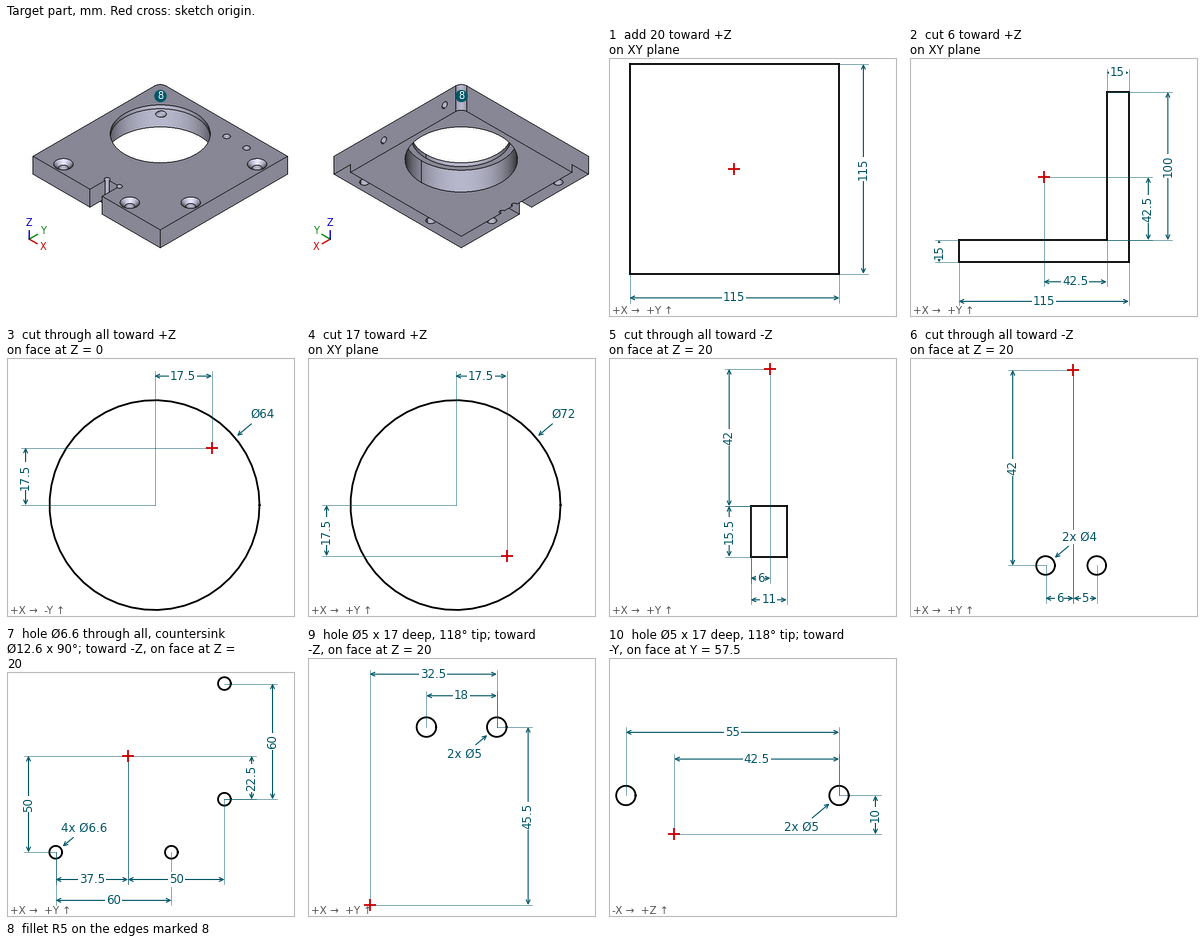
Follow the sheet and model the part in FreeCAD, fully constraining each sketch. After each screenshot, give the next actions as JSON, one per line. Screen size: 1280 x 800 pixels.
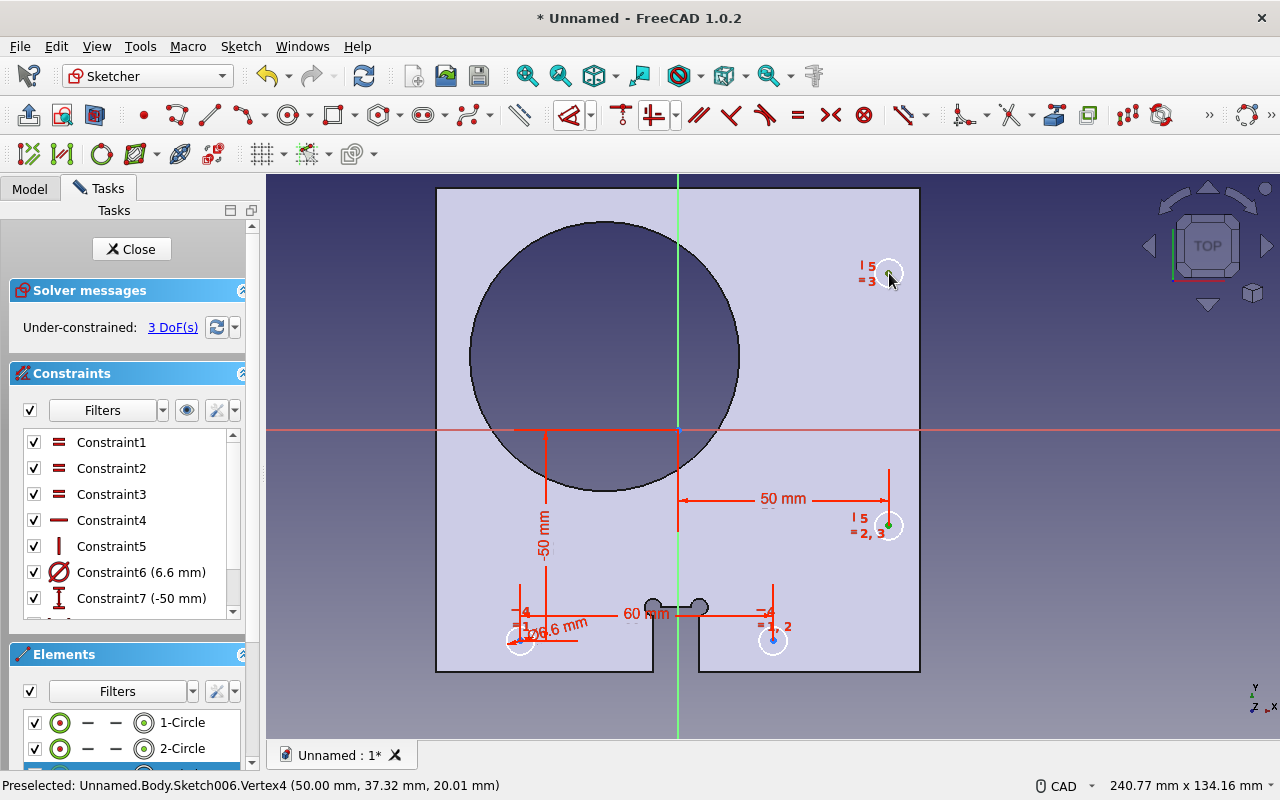
{"action": "key", "text": "i"}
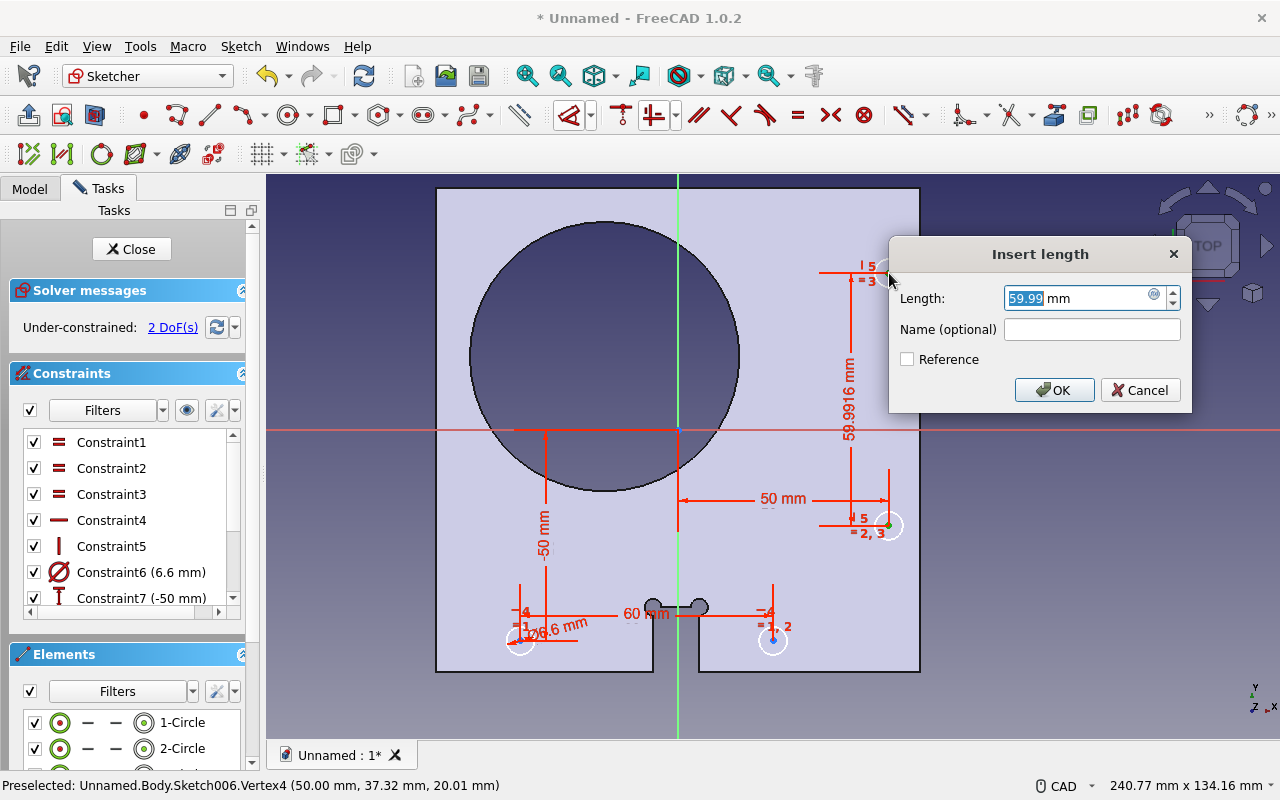
{"action": "type", "text": "60"}
{"action": "key", "text": "Return"}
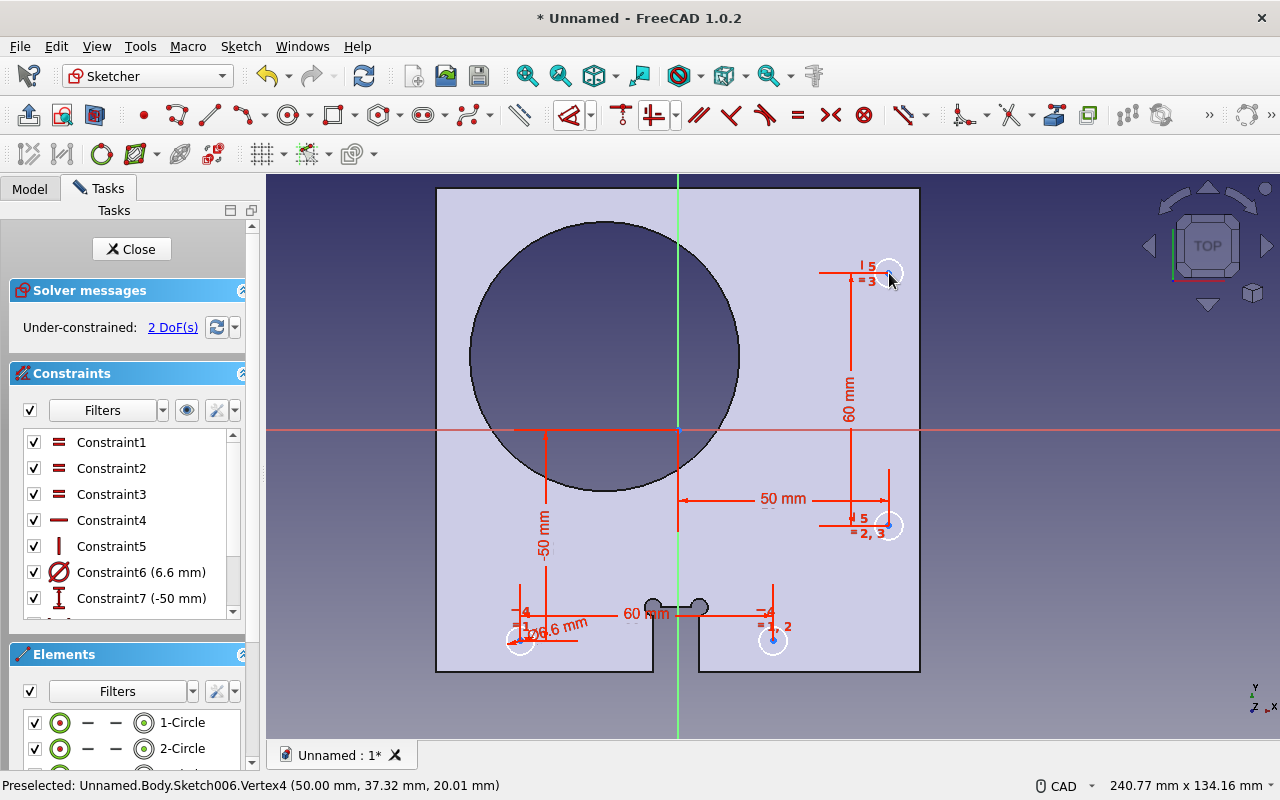
{"action": "left_click", "coordinate": [520, 641]}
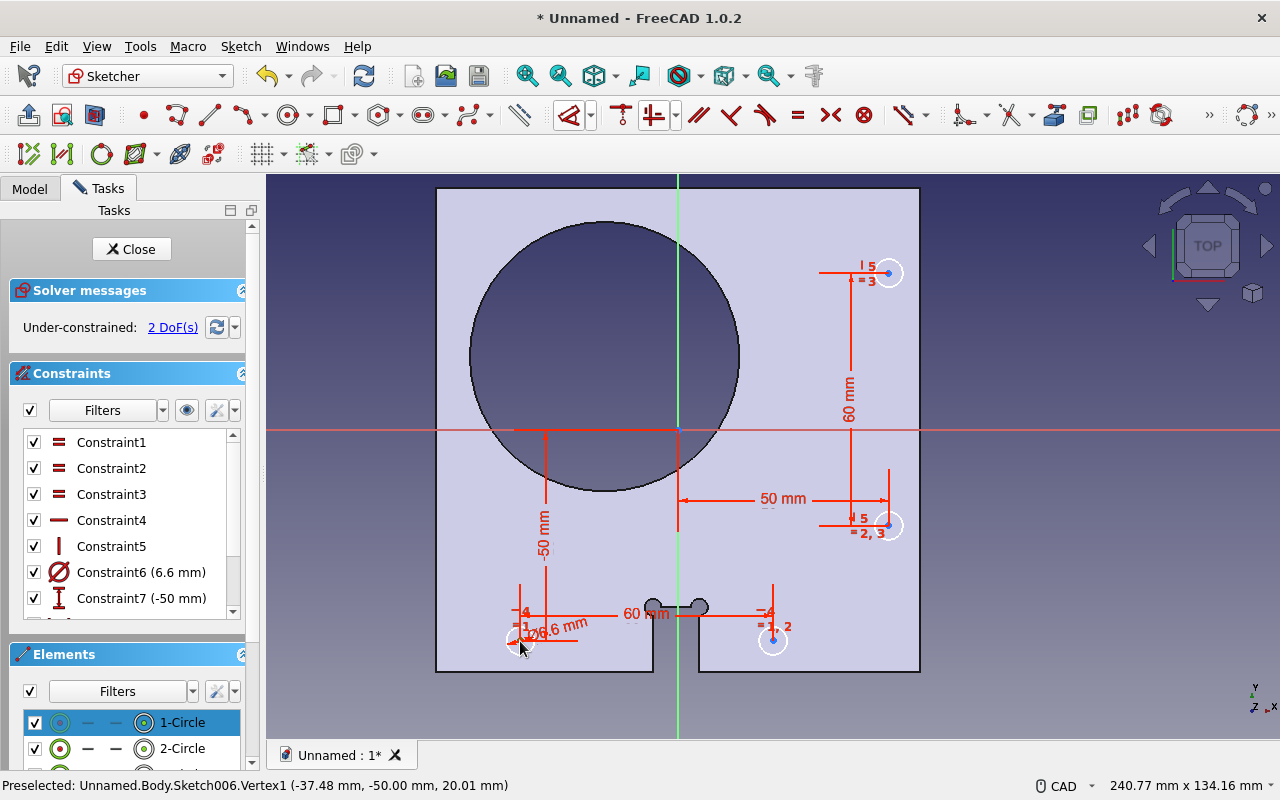
{"action": "left_click", "coordinate": [590, 116]}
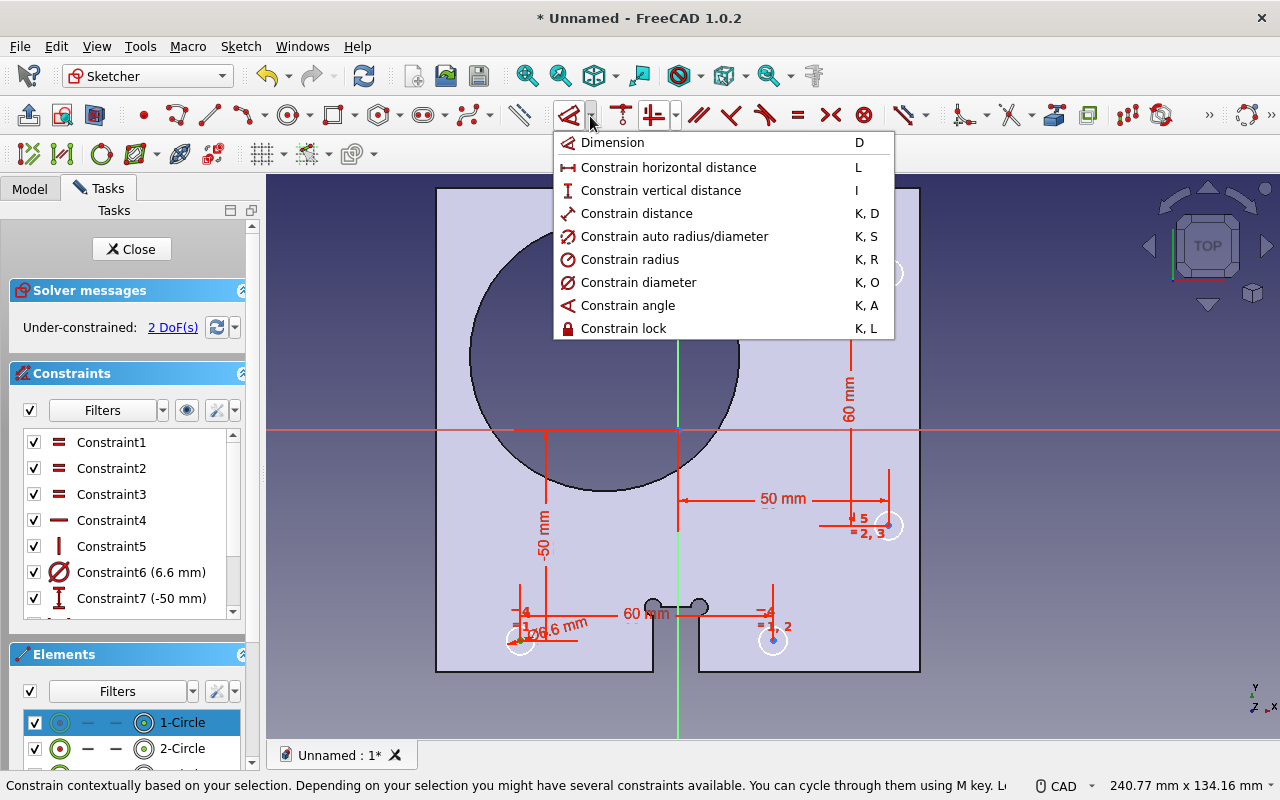
{"action": "left_click", "coordinate": [724, 168]}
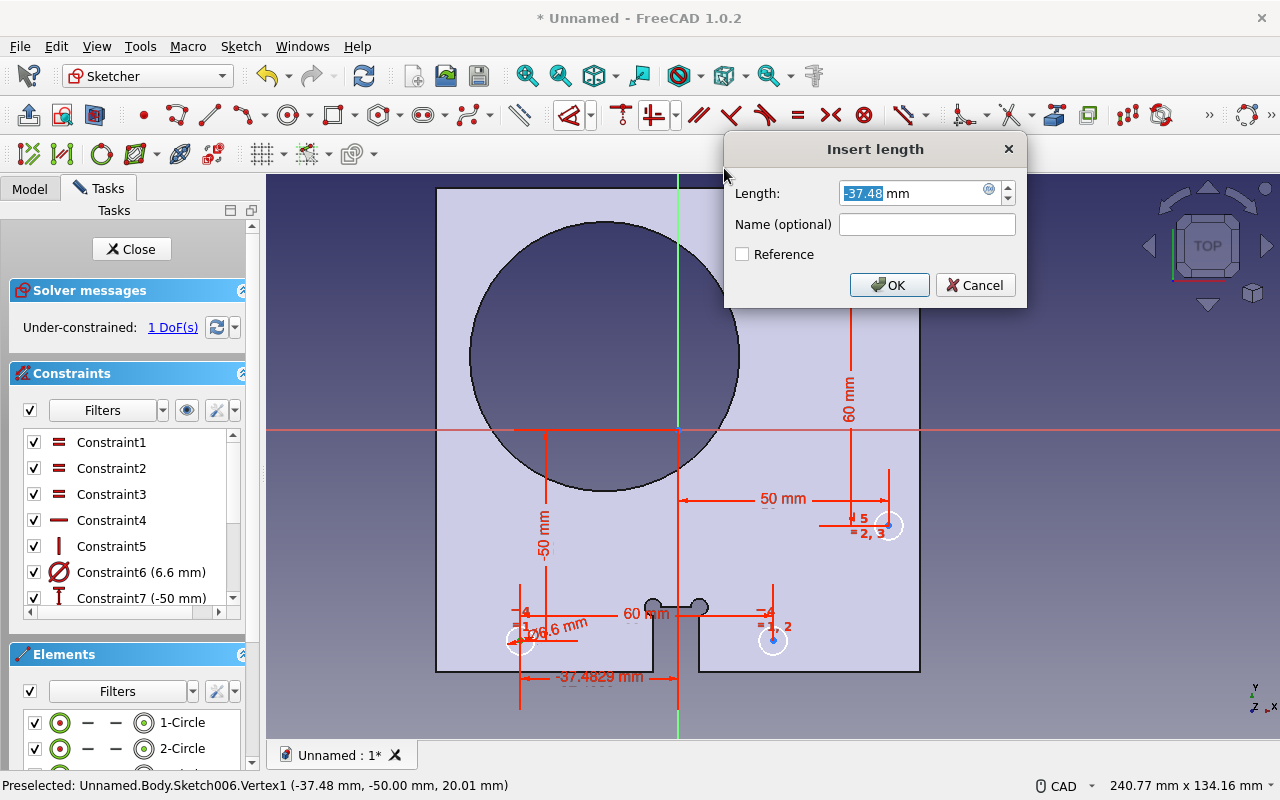
{"action": "type", "text": "-37.5"}
{"action": "key", "text": "Return"}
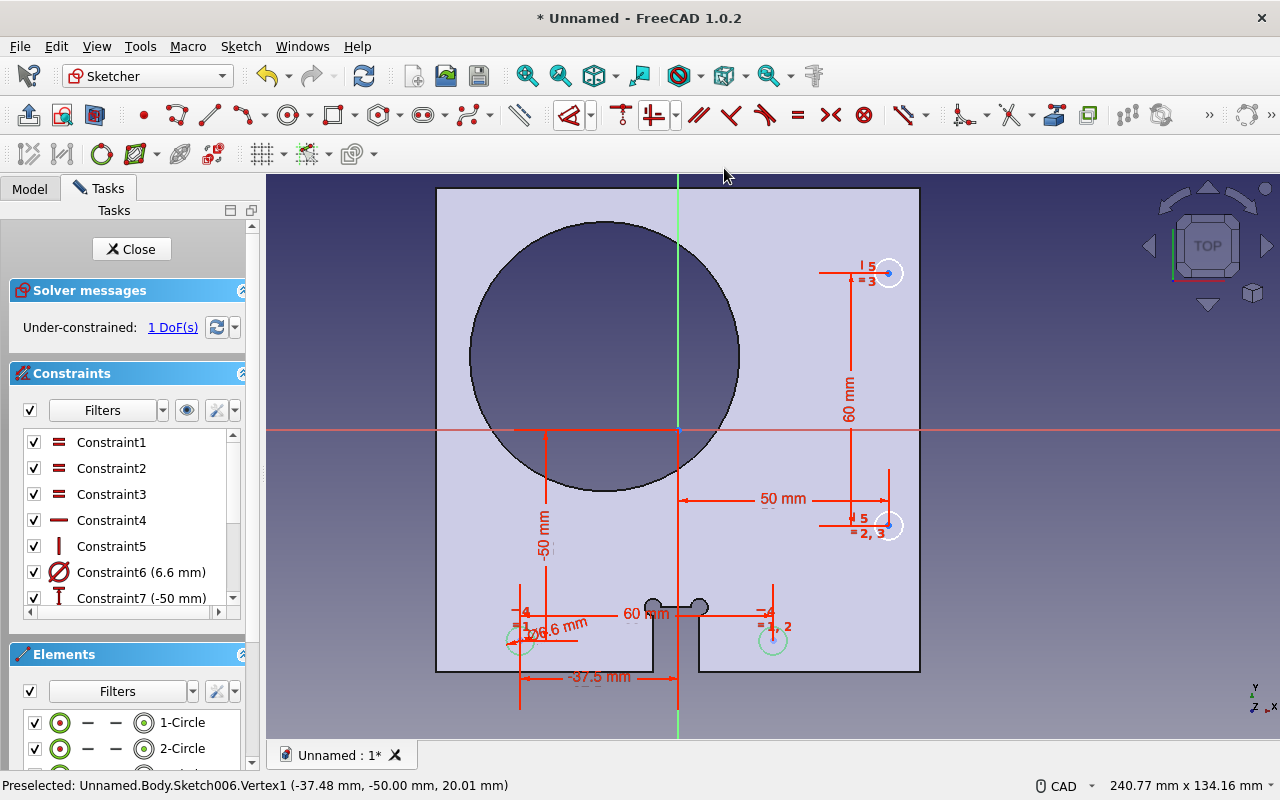
{"action": "left_click", "coordinate": [889, 526]}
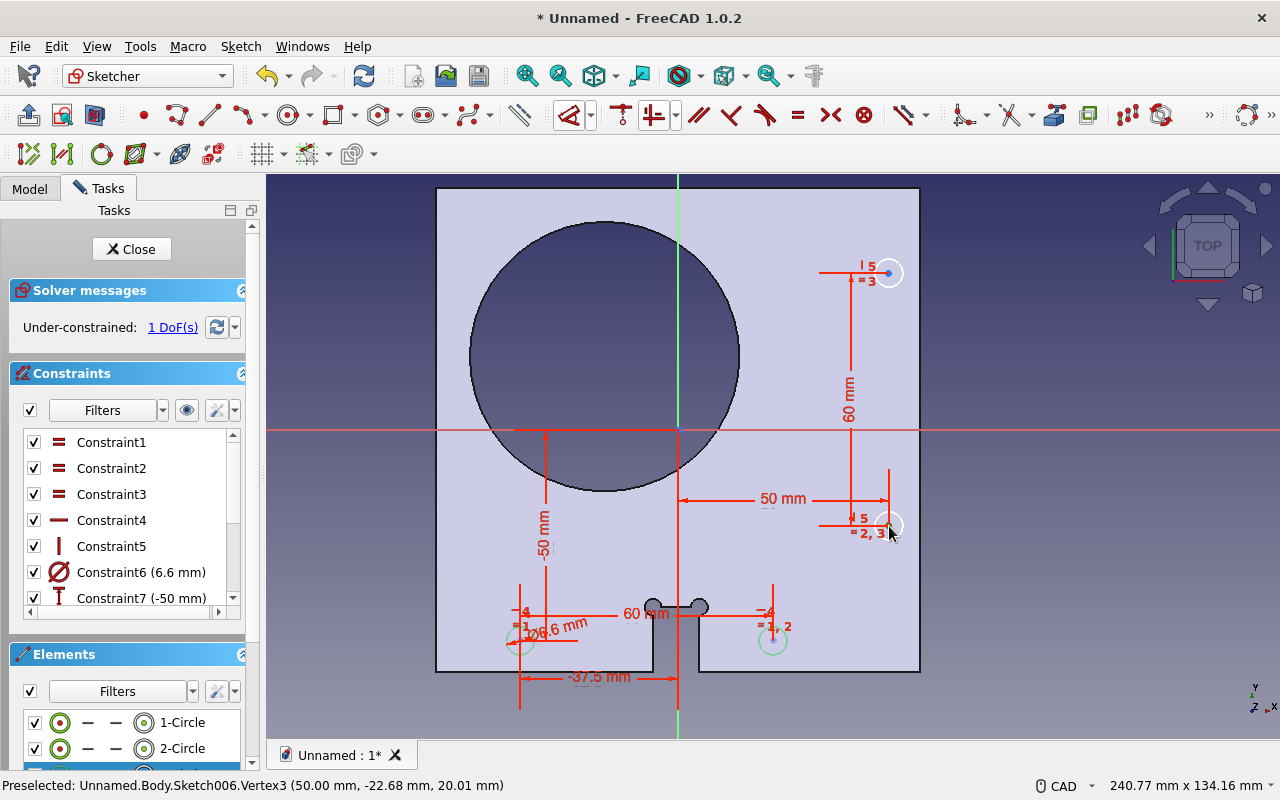
{"action": "key", "text": "i"}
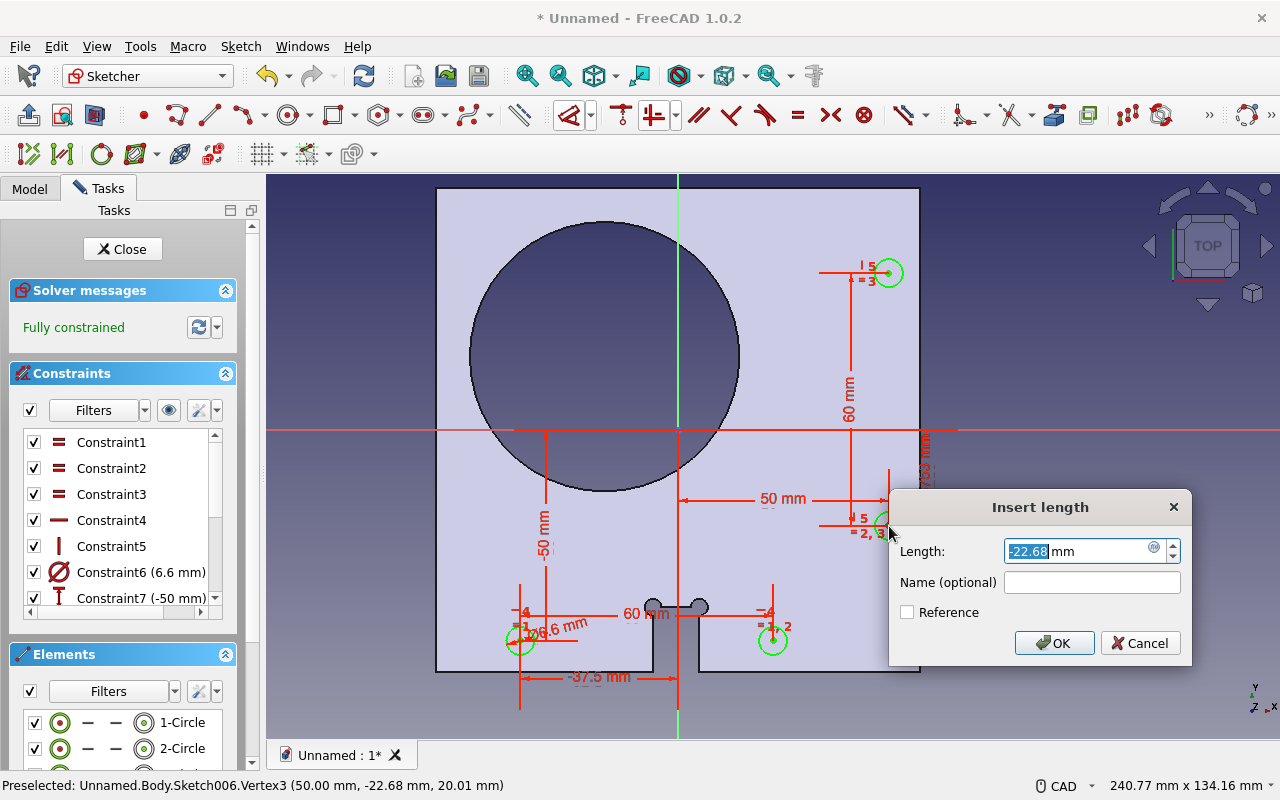
{"action": "type", "text": "-22.5"}
{"action": "key", "text": "Return"}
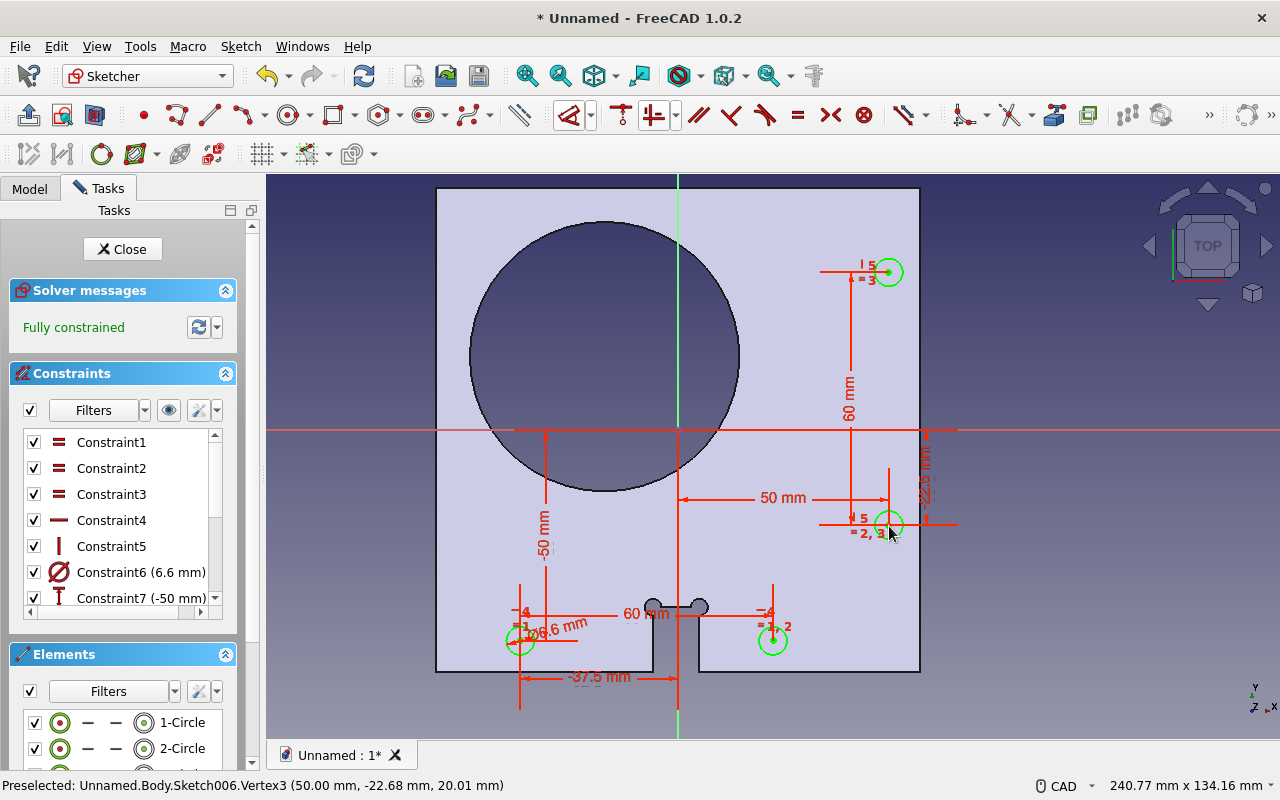
{"action": "left_click", "coordinate": [123, 249]}